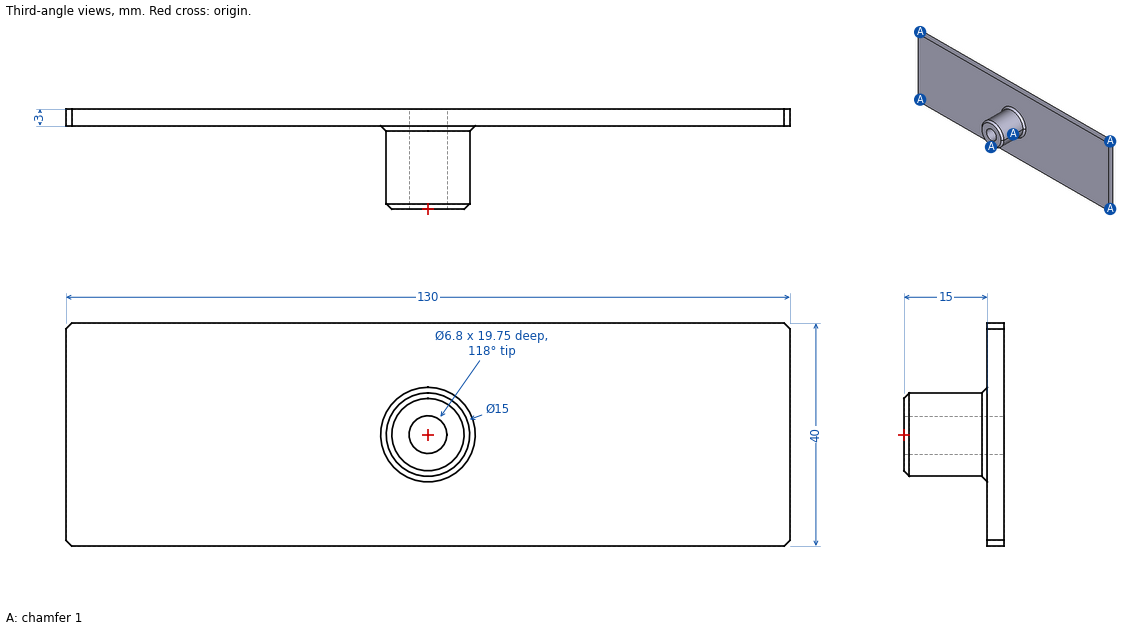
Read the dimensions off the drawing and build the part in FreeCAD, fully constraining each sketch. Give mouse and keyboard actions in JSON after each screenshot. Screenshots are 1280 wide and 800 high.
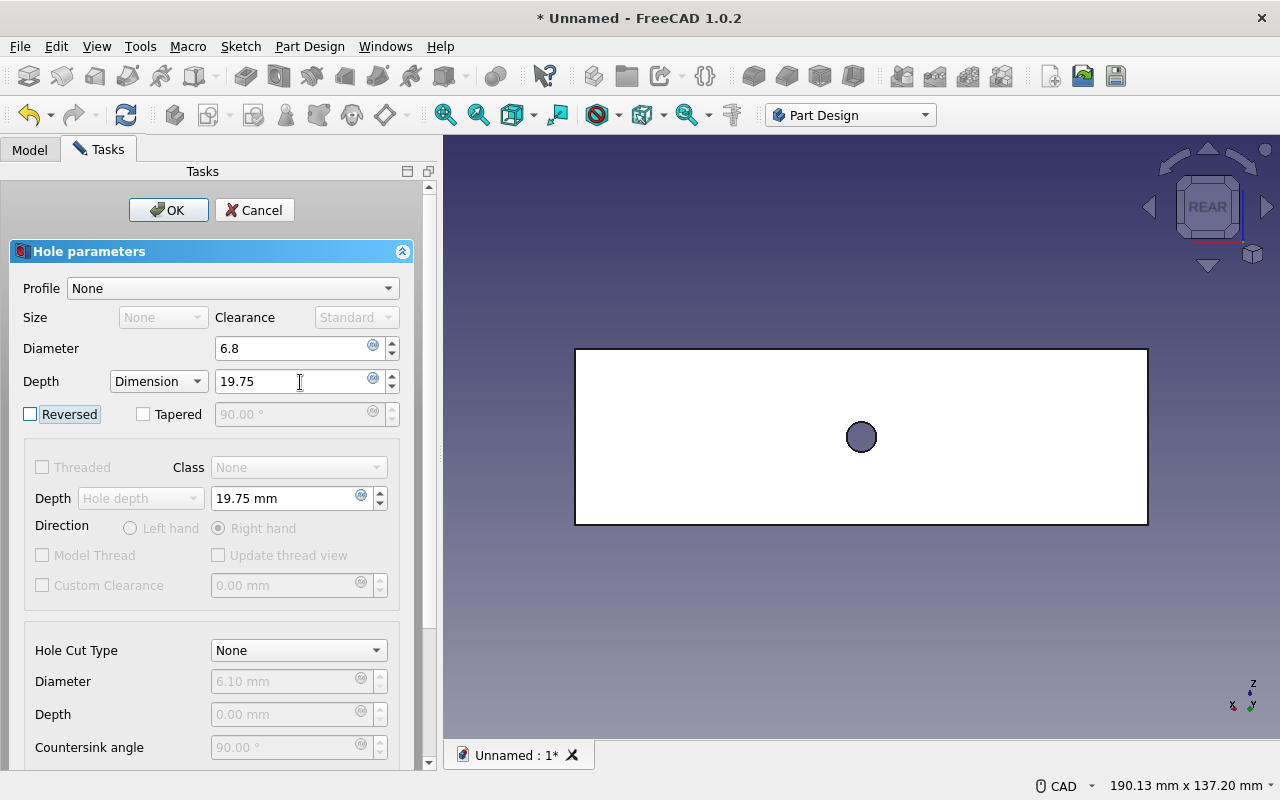
{"action": "left_click", "coordinate": [169, 210]}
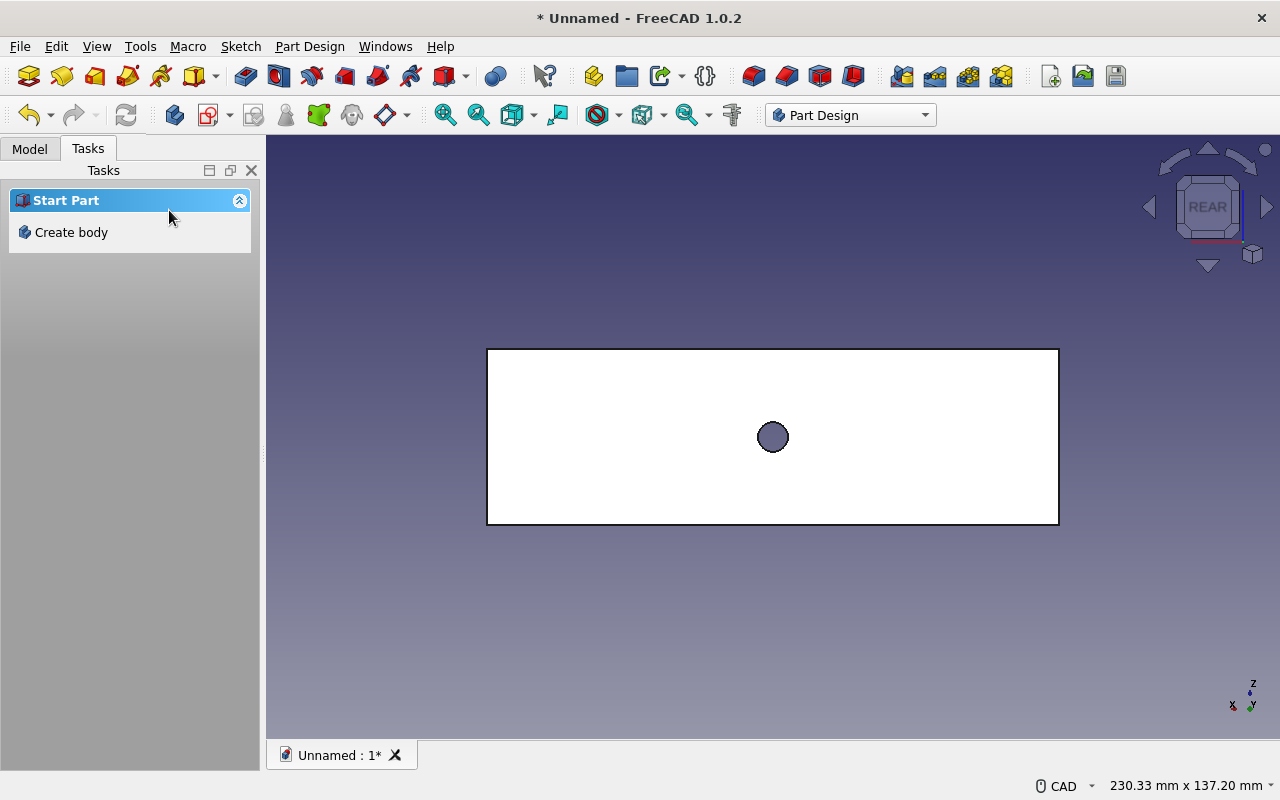
{"action": "key", "text": "0"}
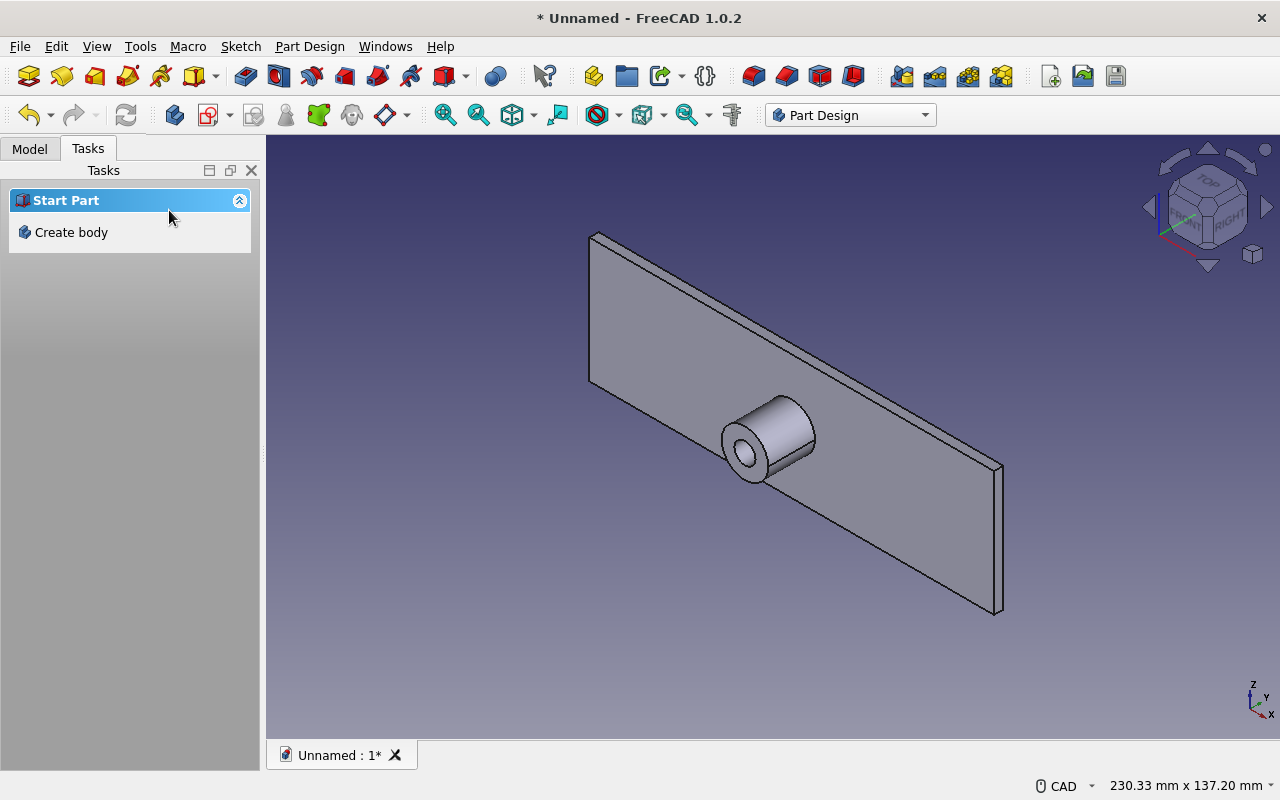
{"action": "left_click", "coordinate": [726, 425]}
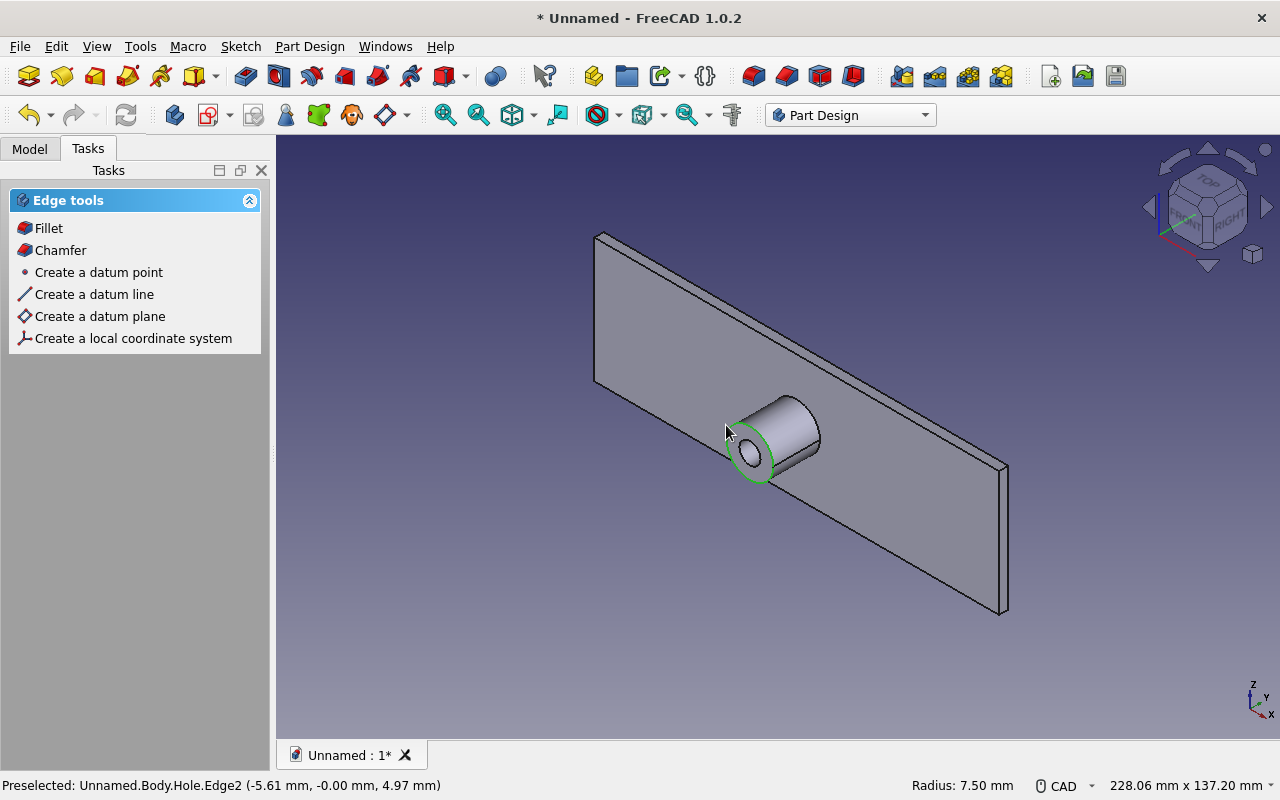
{"action": "left_click", "coordinate": [1005, 467], "text": "ctrl"}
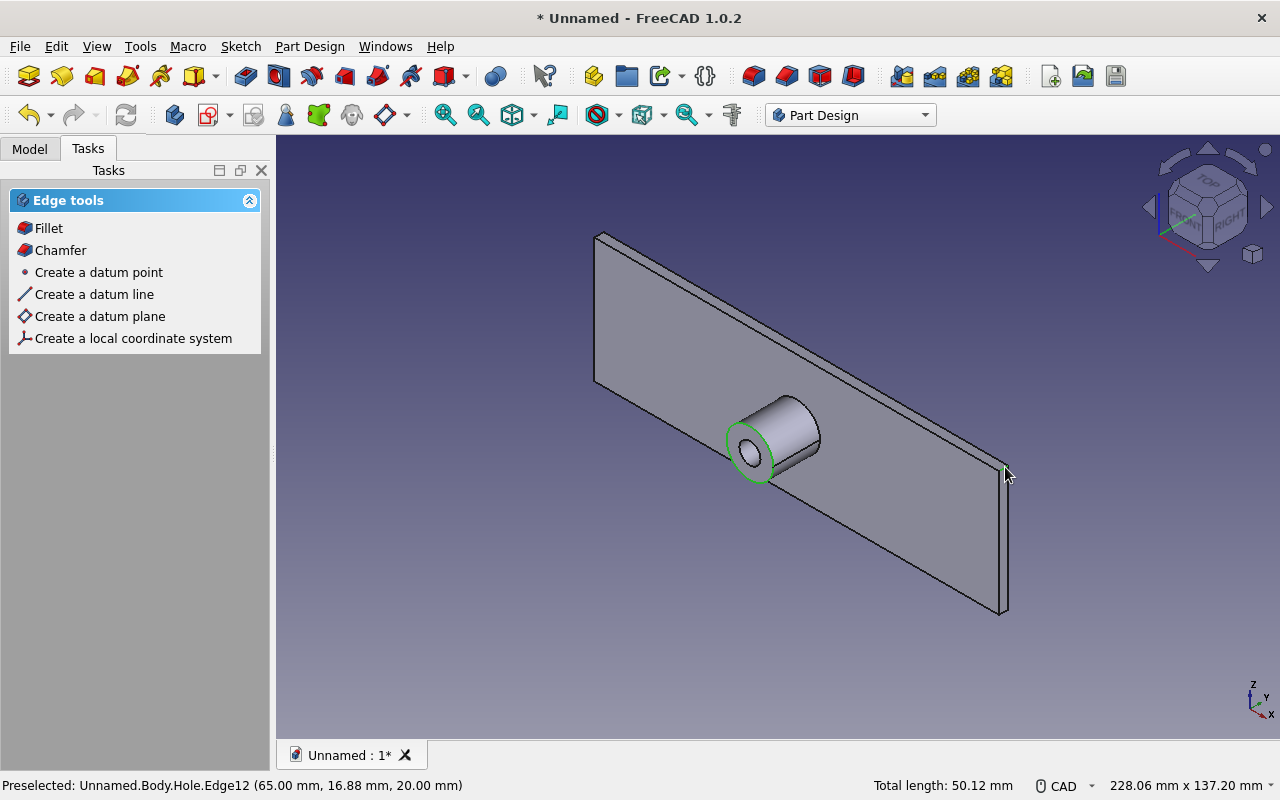
{"action": "key", "text": "2"}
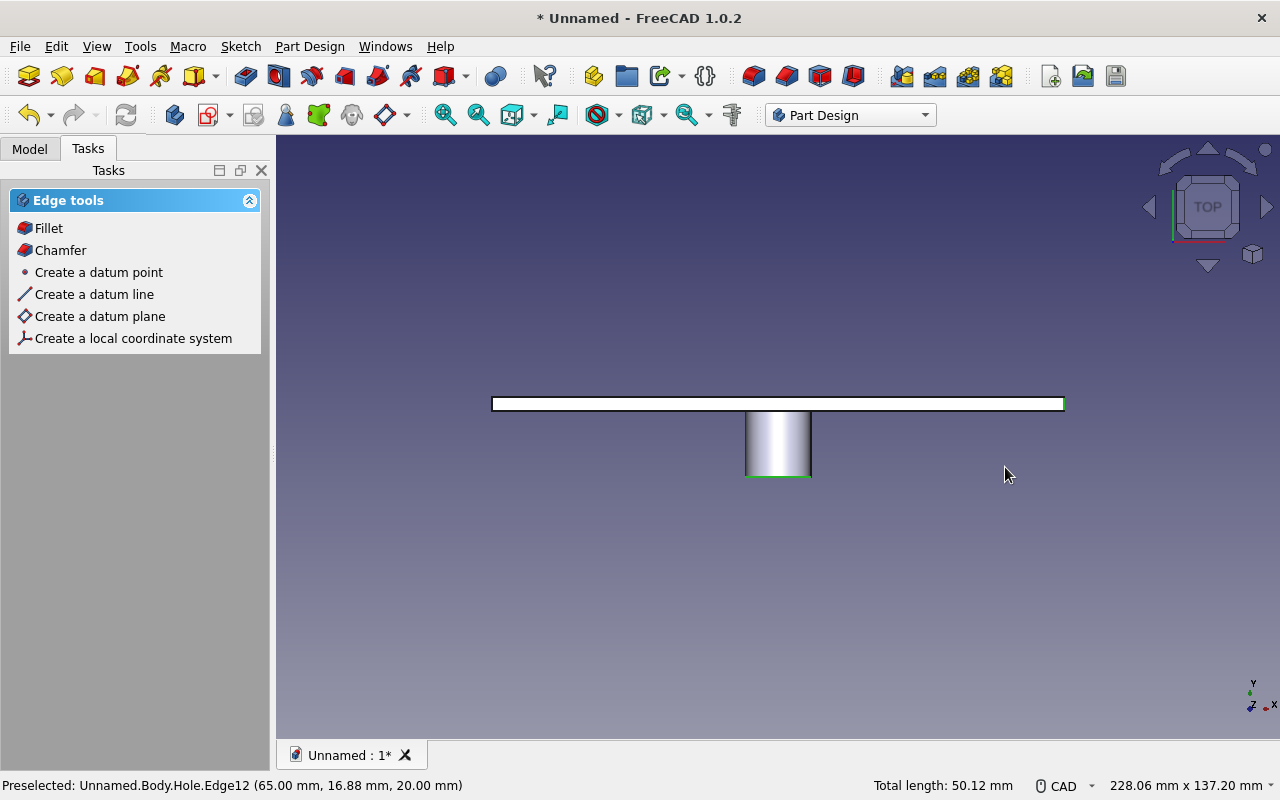
{"action": "left_click", "coordinate": [492, 403], "text": "ctrl"}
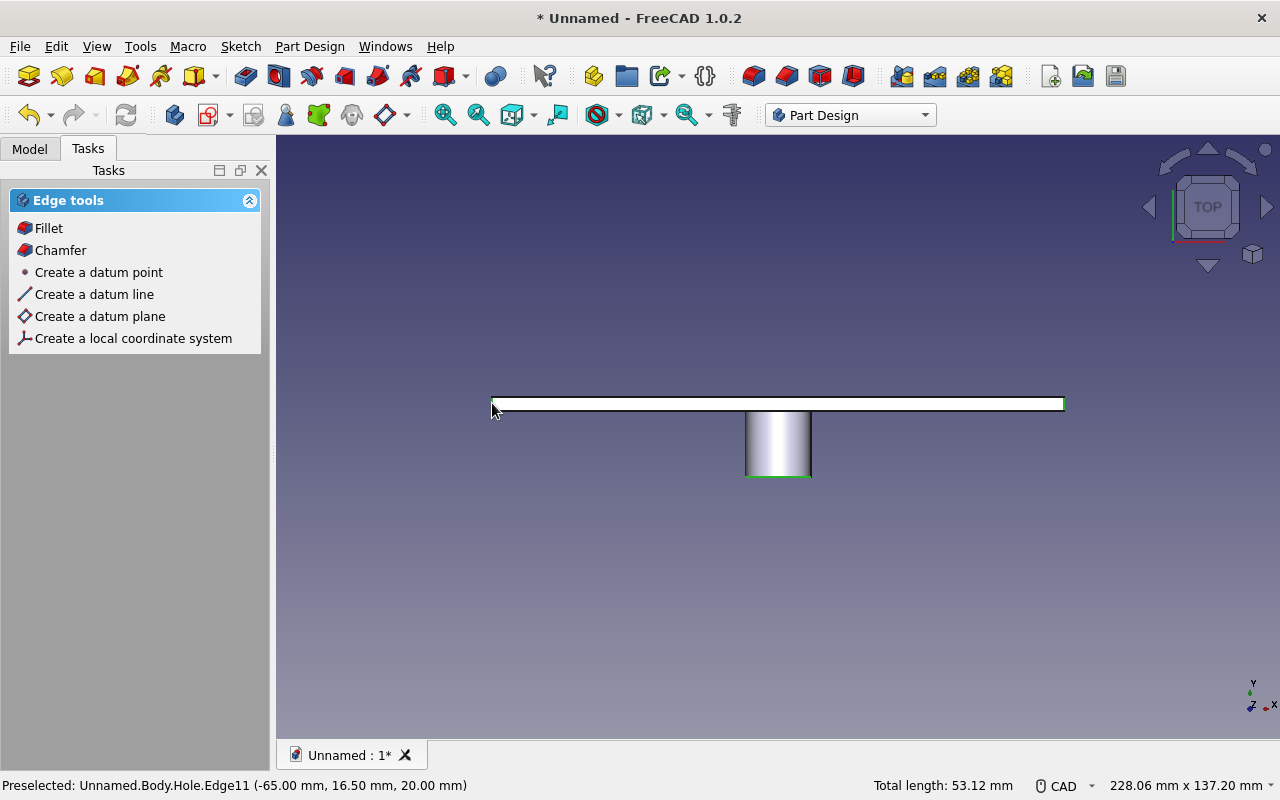
{"action": "key", "text": "1"}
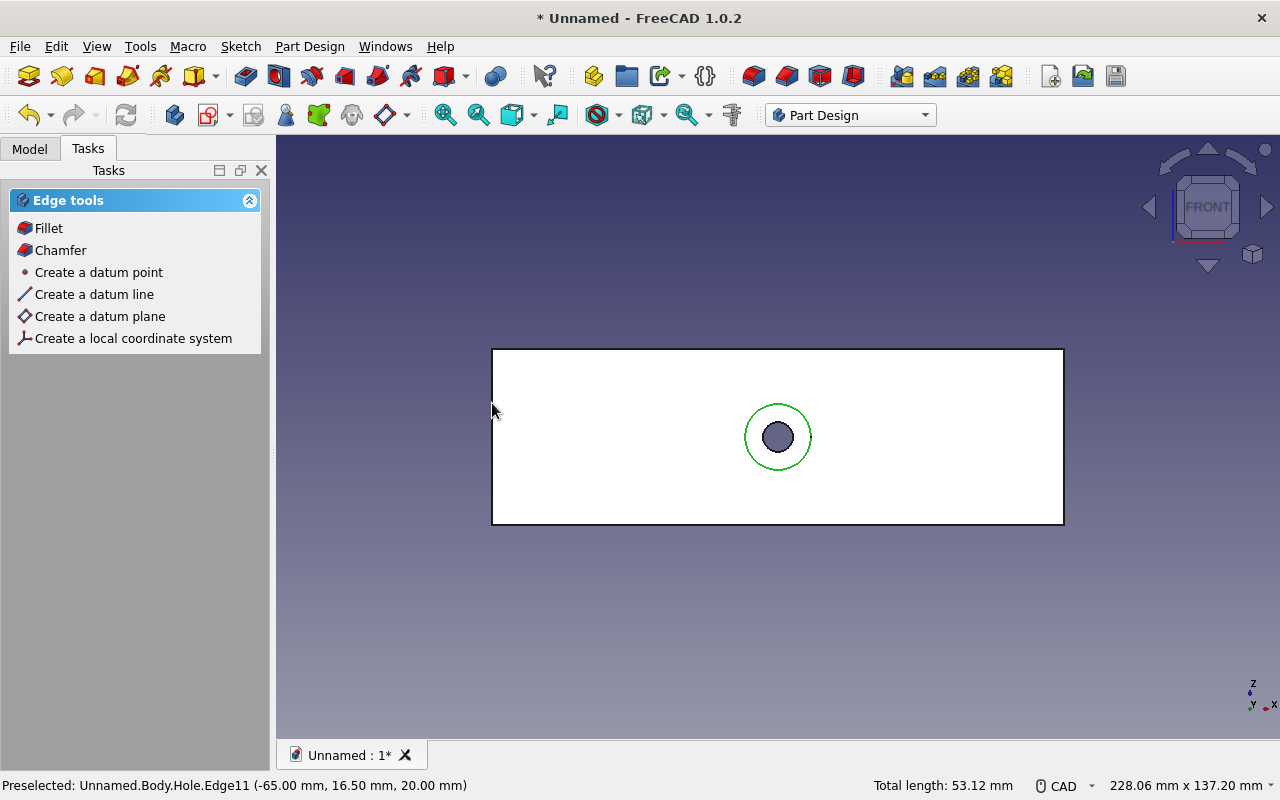
{"action": "key", "text": "3"}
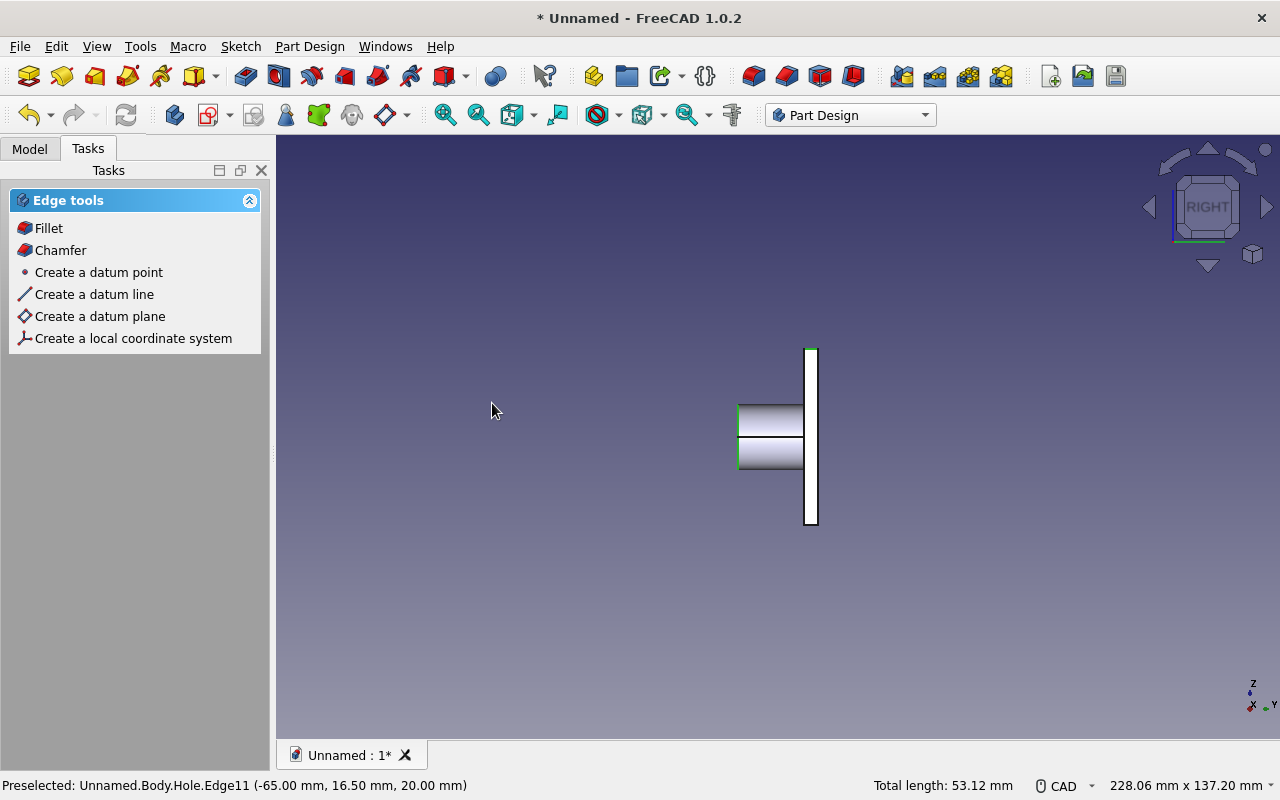
{"action": "left_click", "coordinate": [446, 116]}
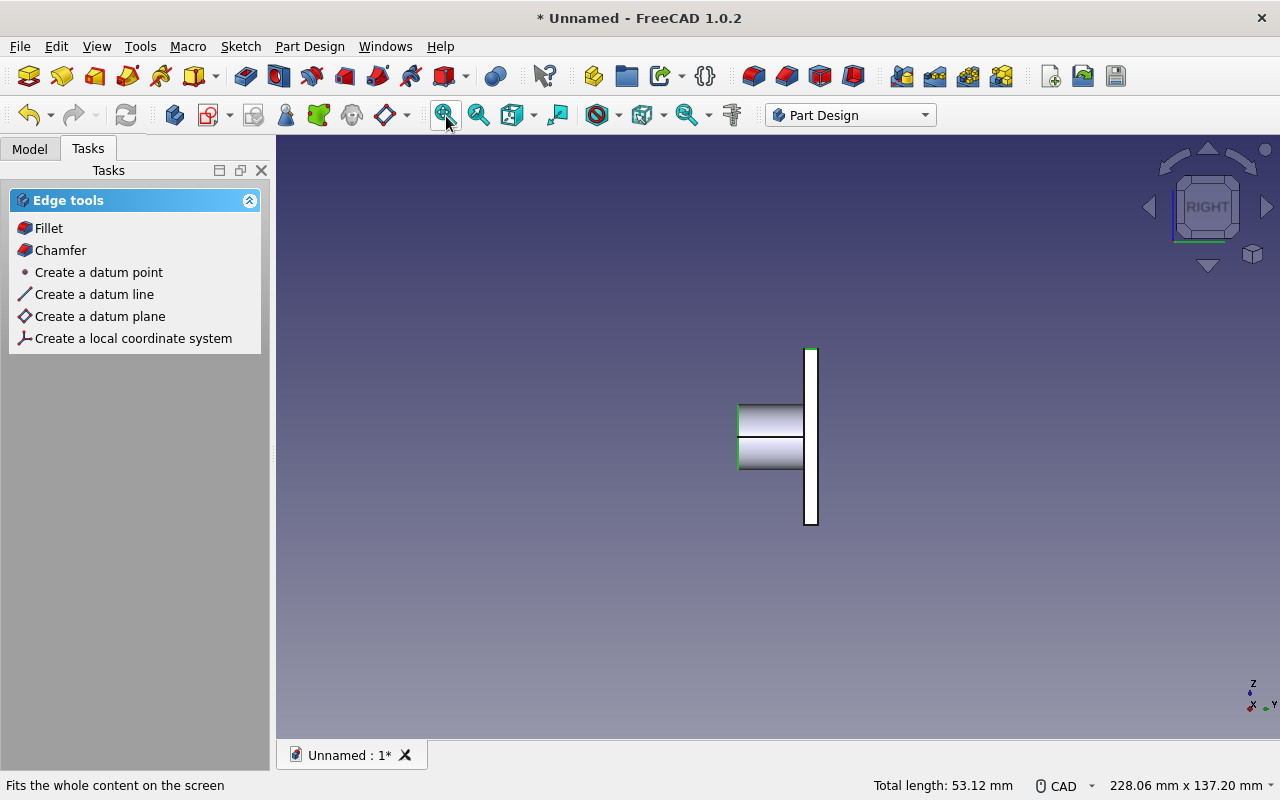
{"action": "left_click", "coordinate": [811, 524], "text": "ctrl"}